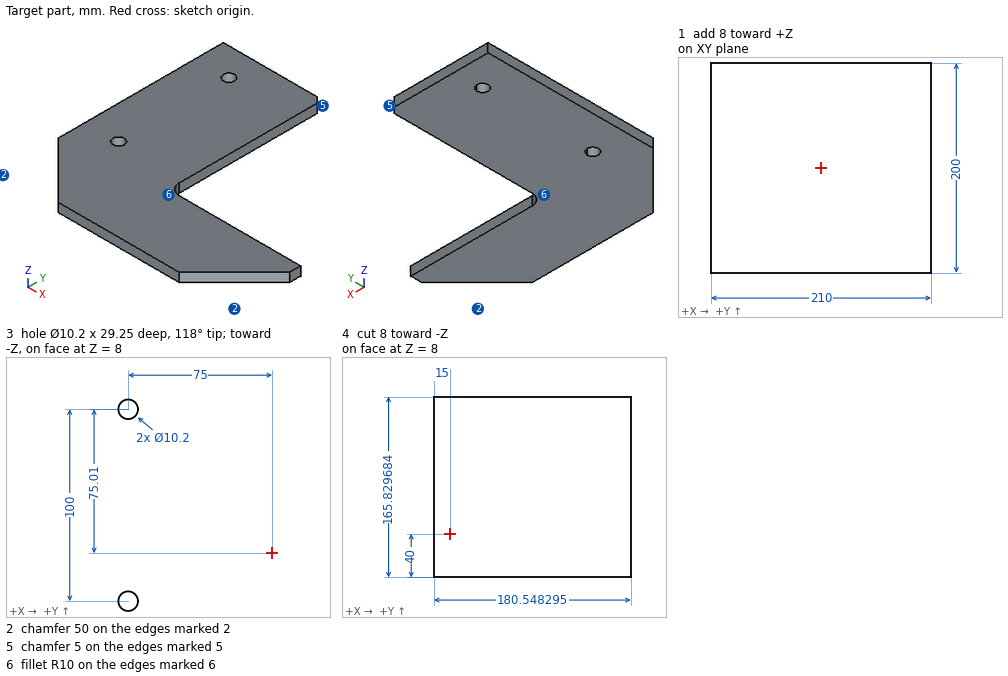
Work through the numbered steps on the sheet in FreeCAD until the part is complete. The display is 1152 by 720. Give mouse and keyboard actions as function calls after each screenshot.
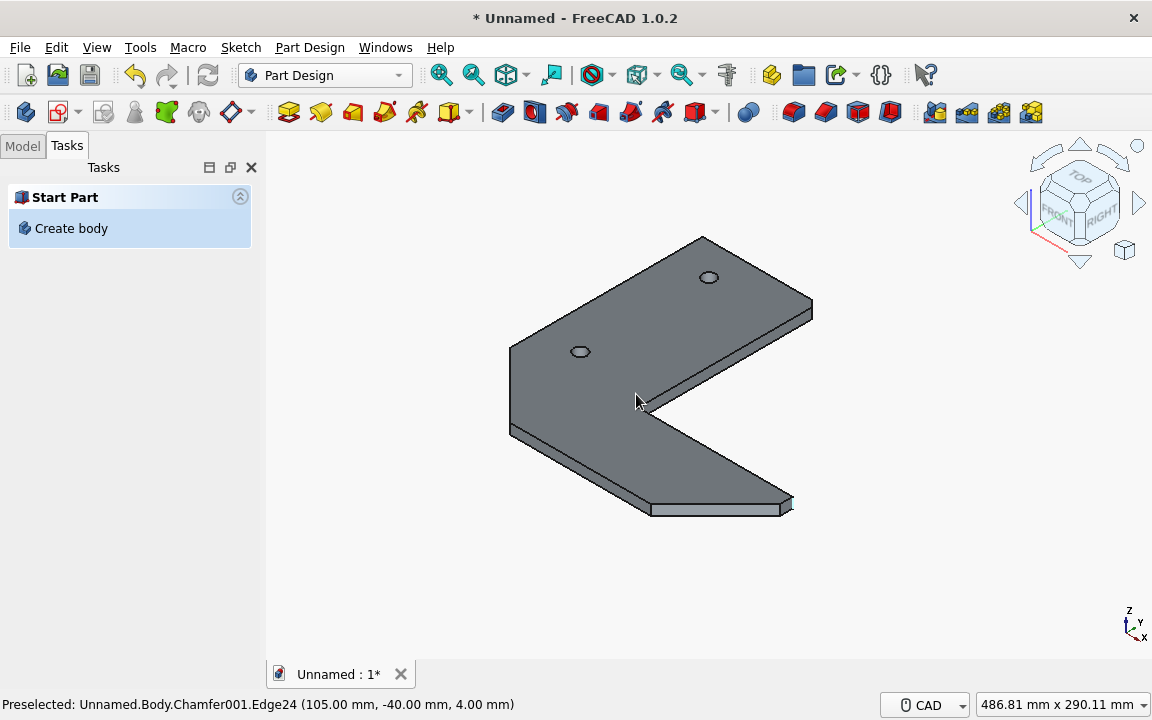
scroll(638, 413, up, 6)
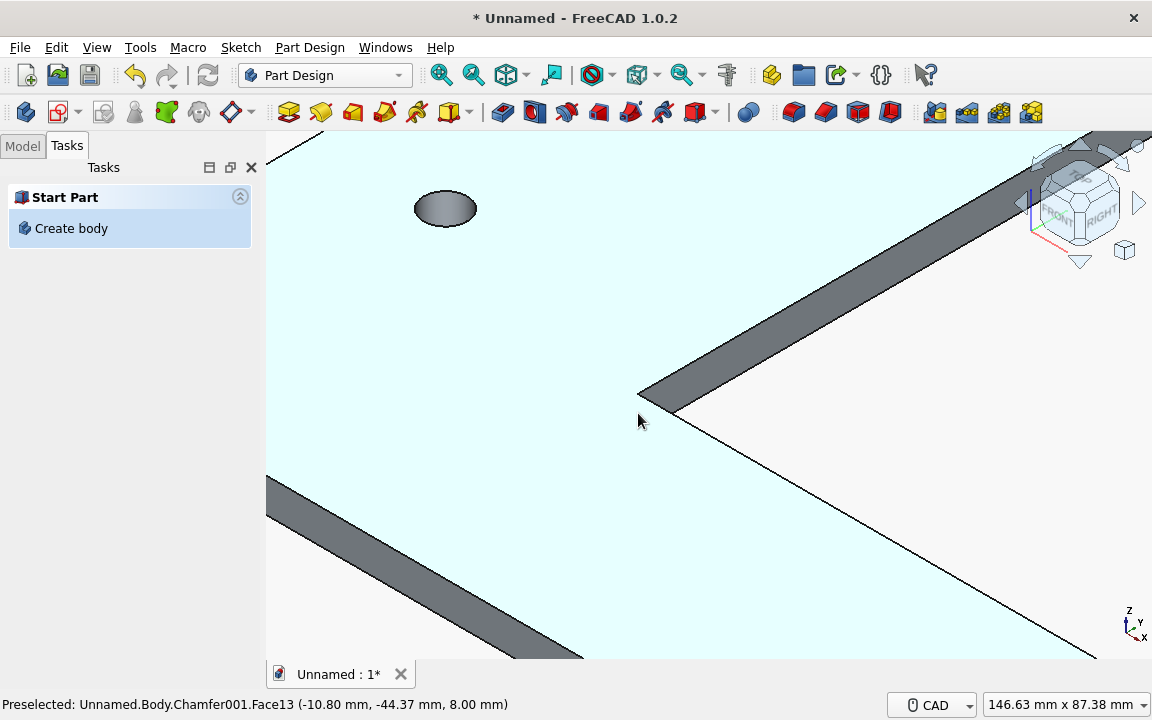
key(v)
key(f)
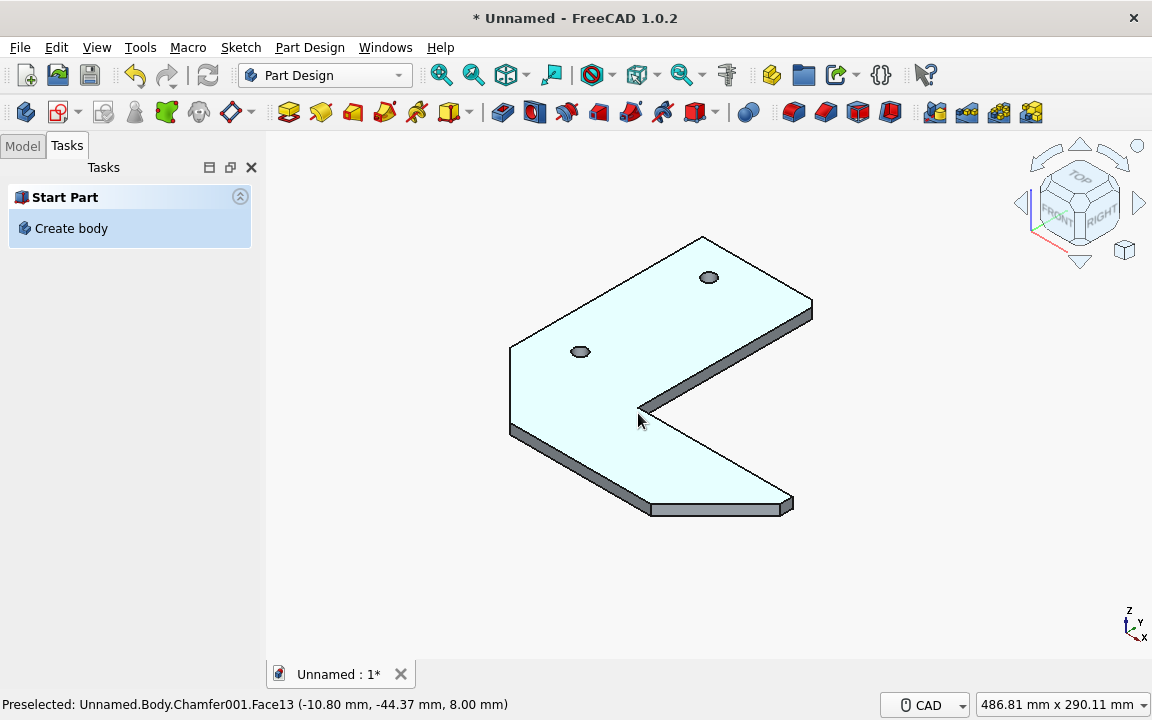
key(2)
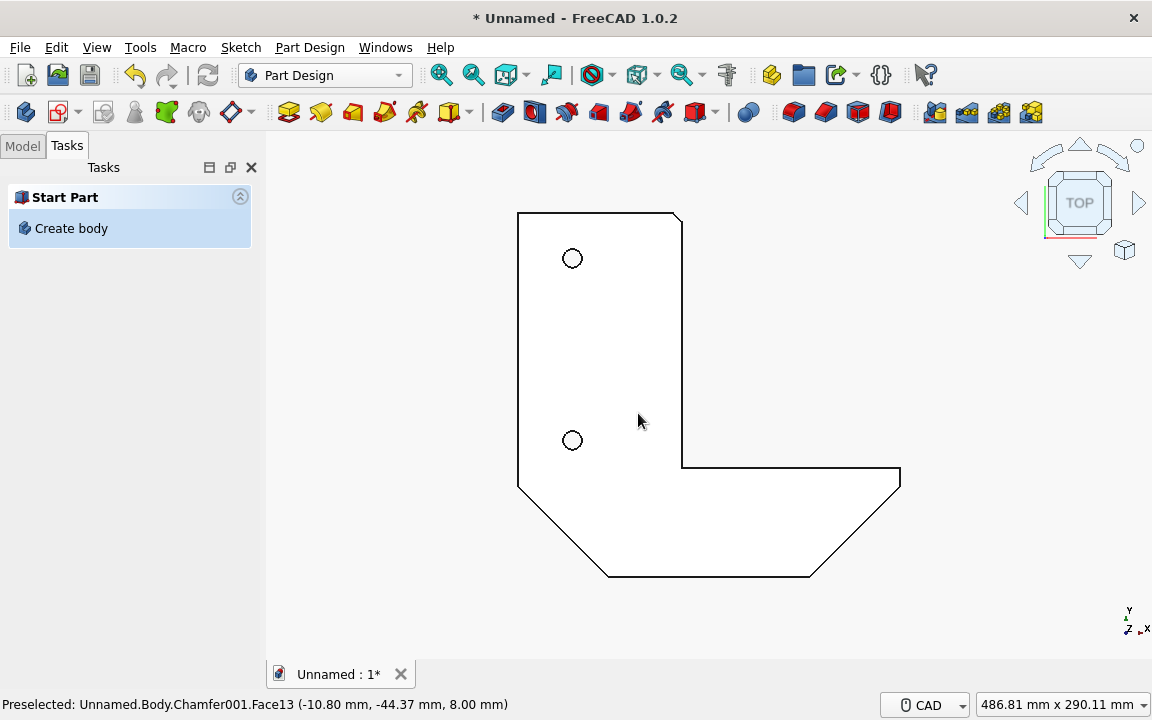
scroll(682, 467, up, 6)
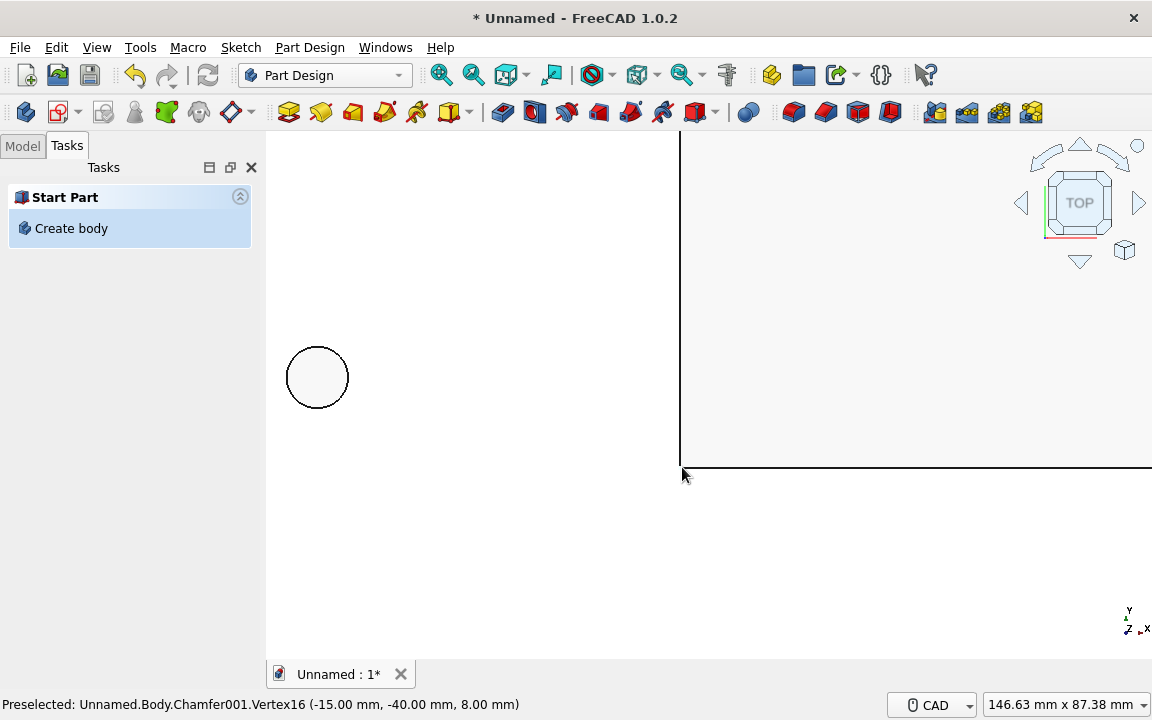
click(442, 76)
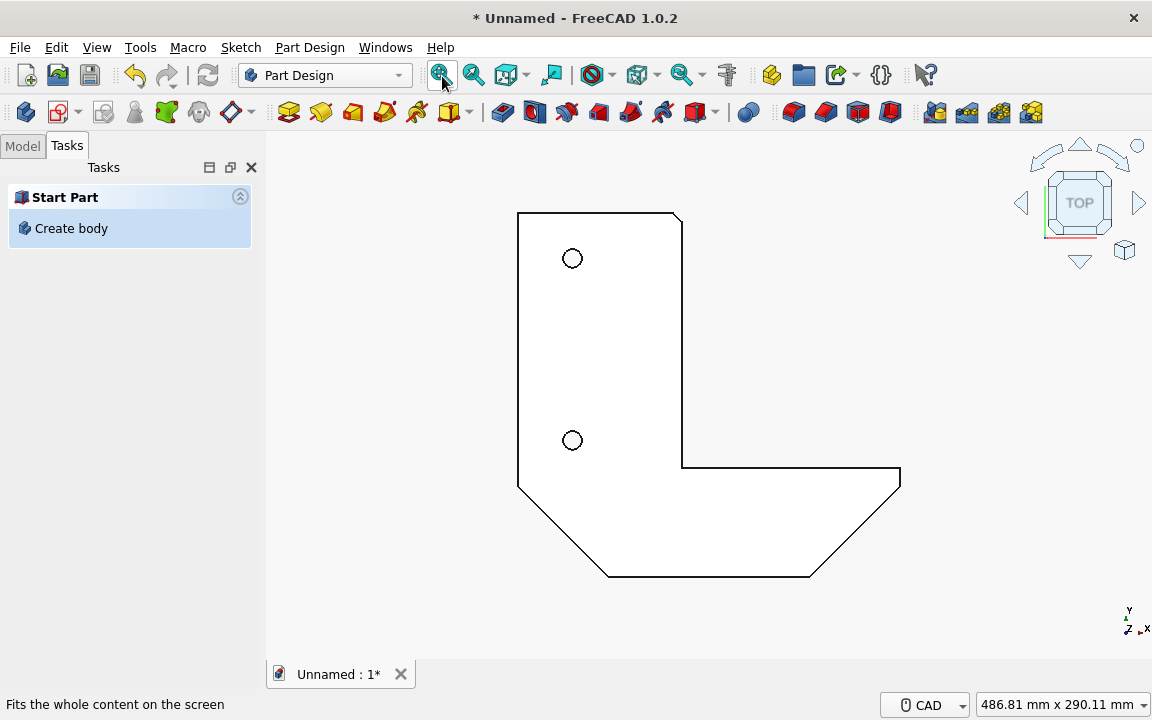
key(1)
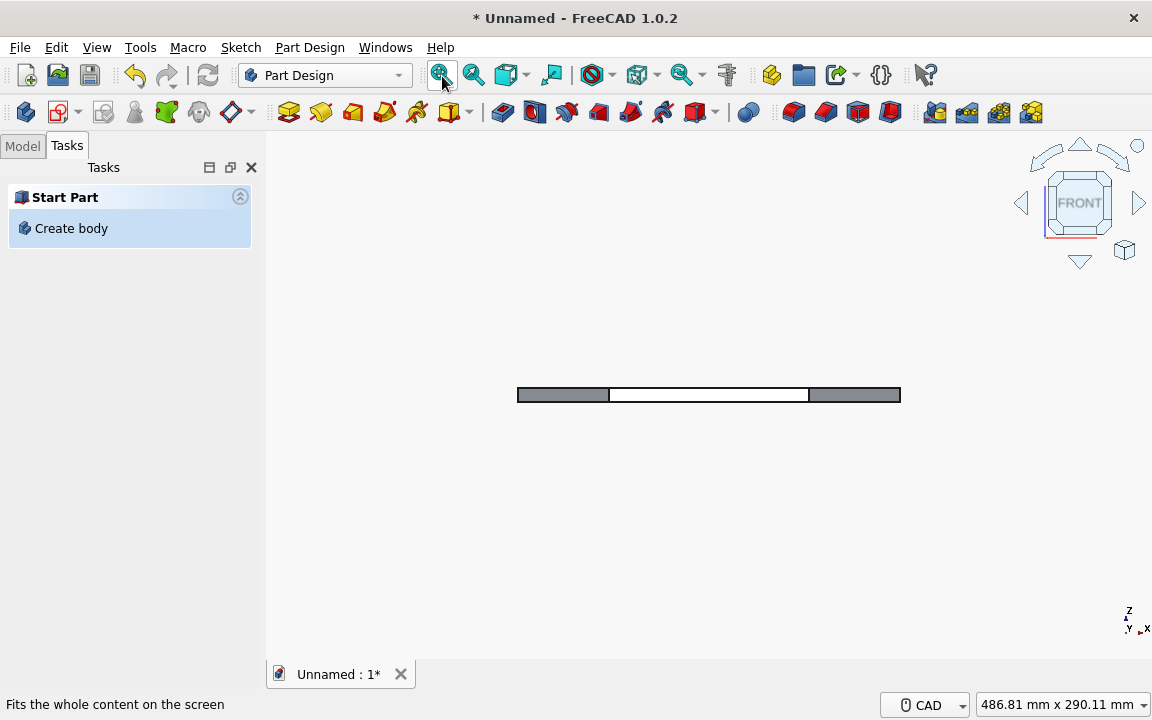
key(v)
key(f)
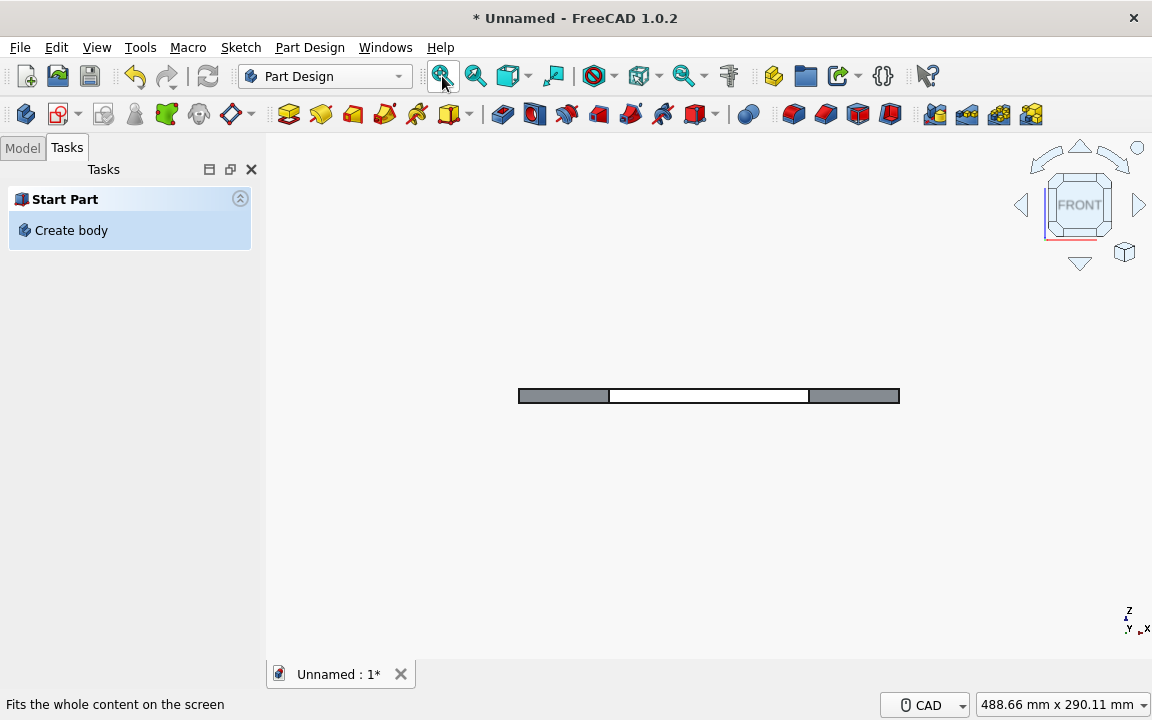
scroll(682, 395, up, 6)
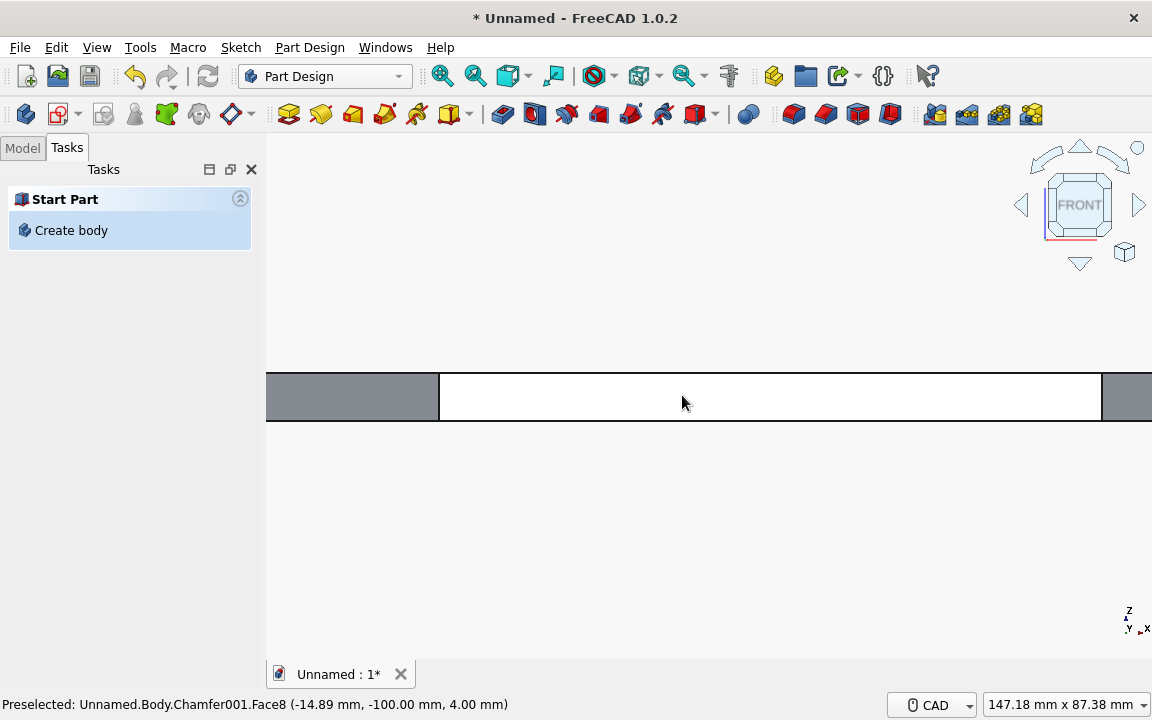
key(v)
key(f)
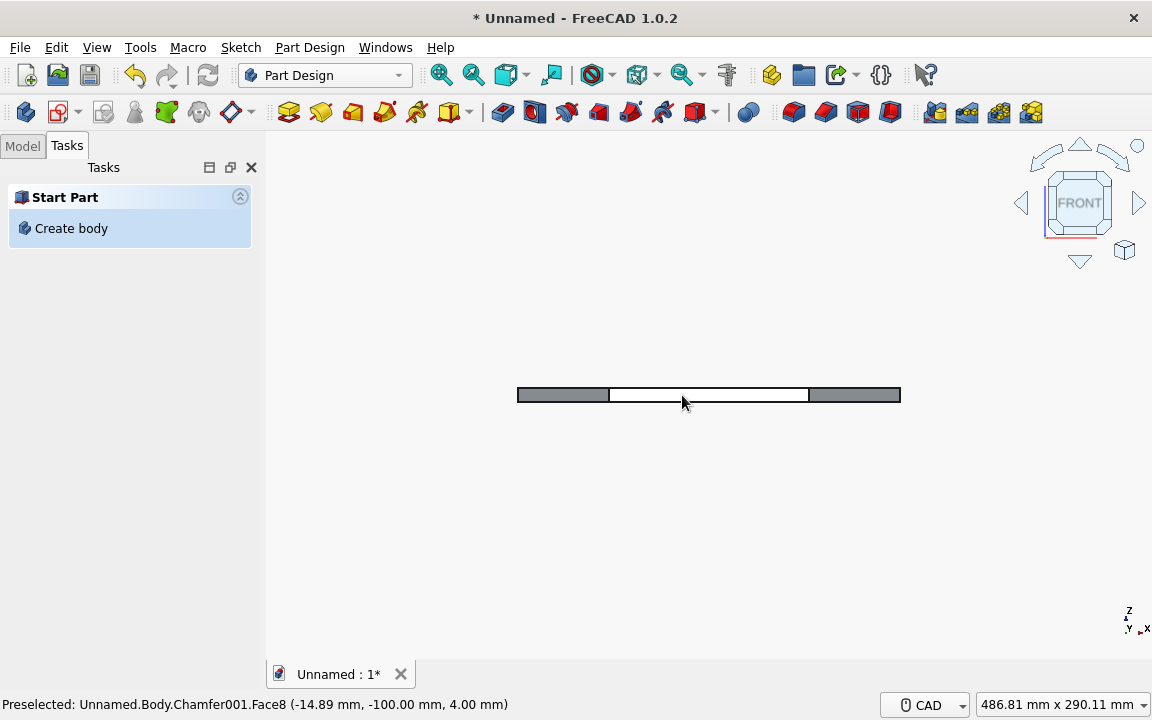
key(3)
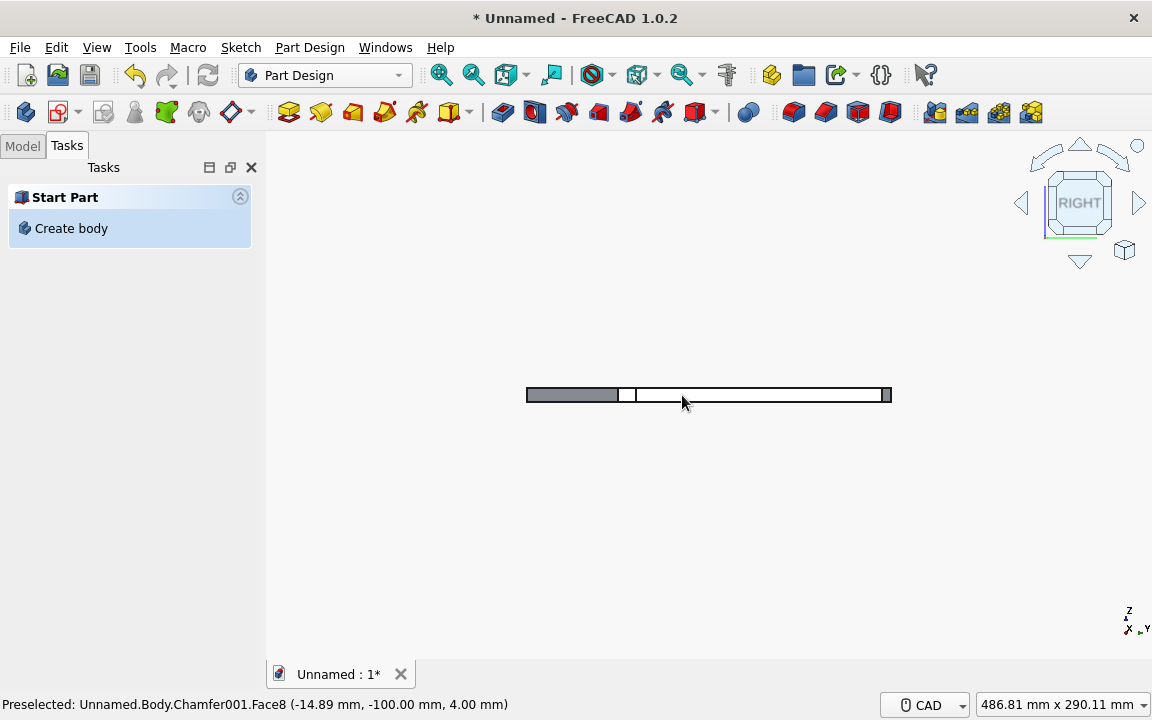
key(v)
key(f)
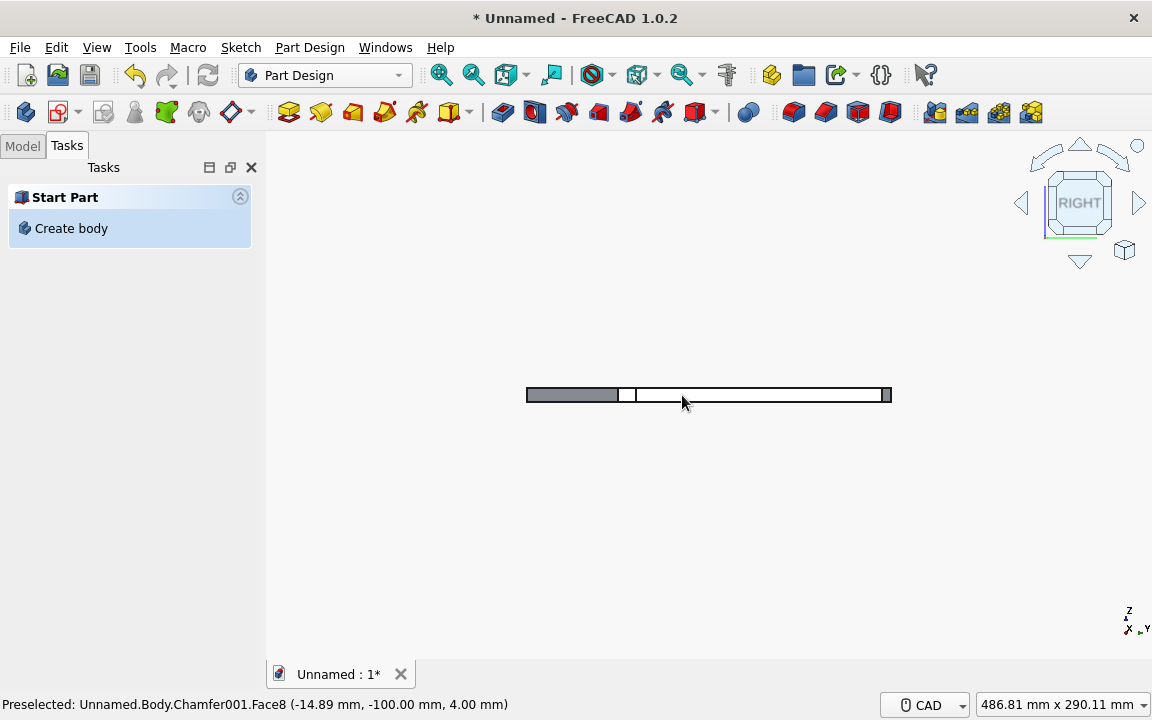
scroll(636, 394, up, 6)